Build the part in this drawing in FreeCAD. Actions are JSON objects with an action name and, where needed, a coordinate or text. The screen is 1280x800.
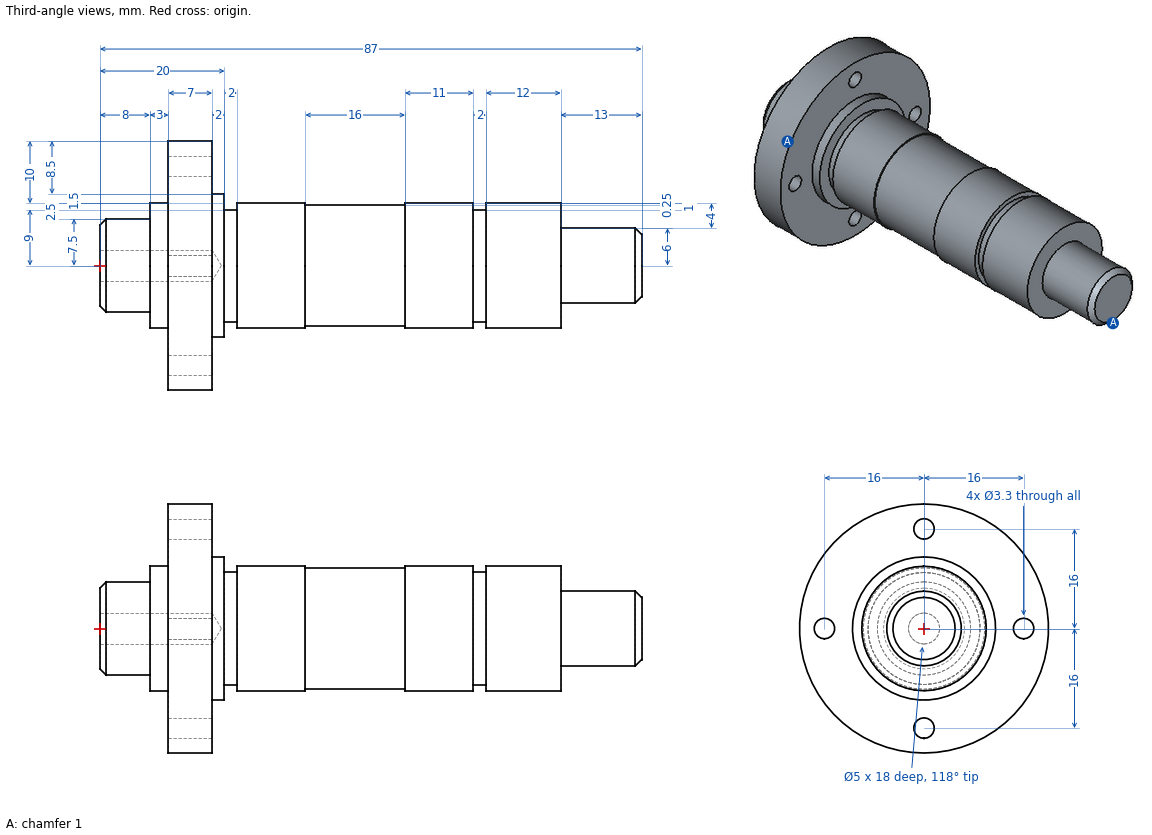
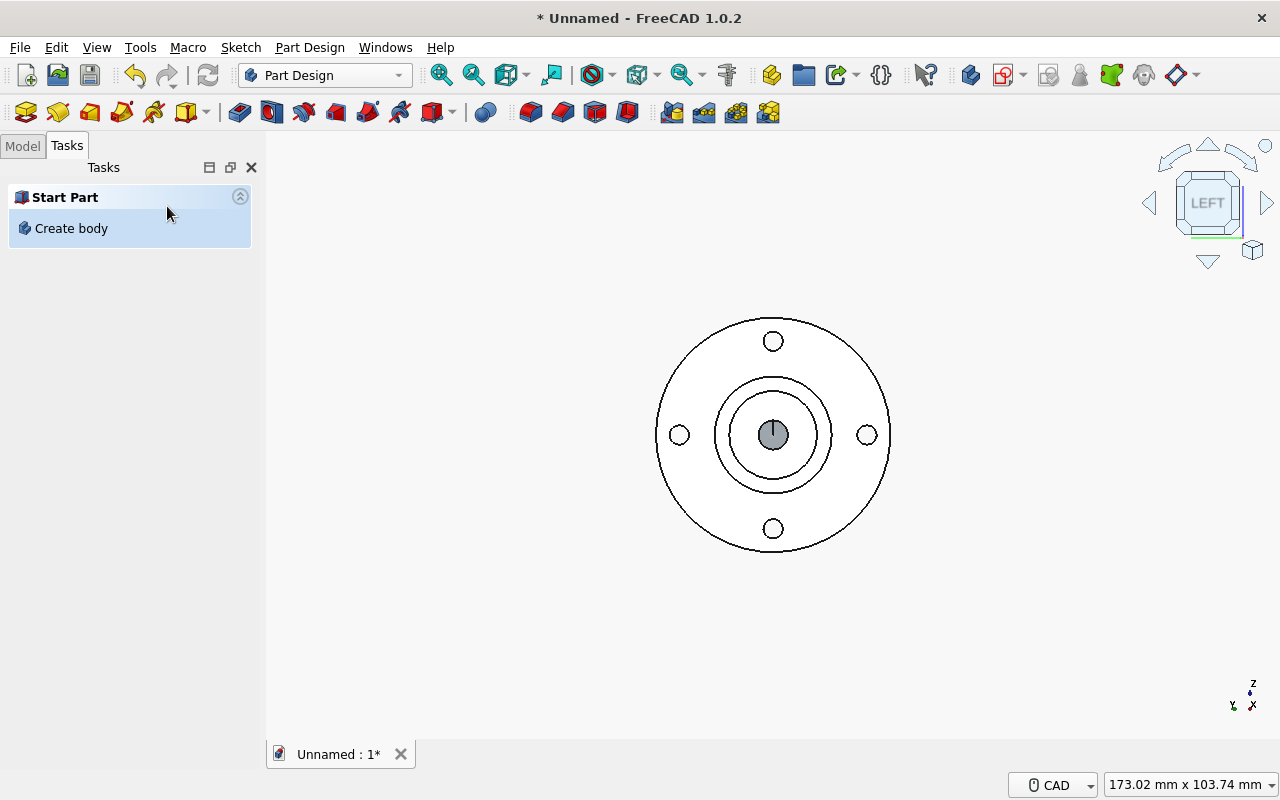
{"action": "left_click", "coordinate": [442, 76]}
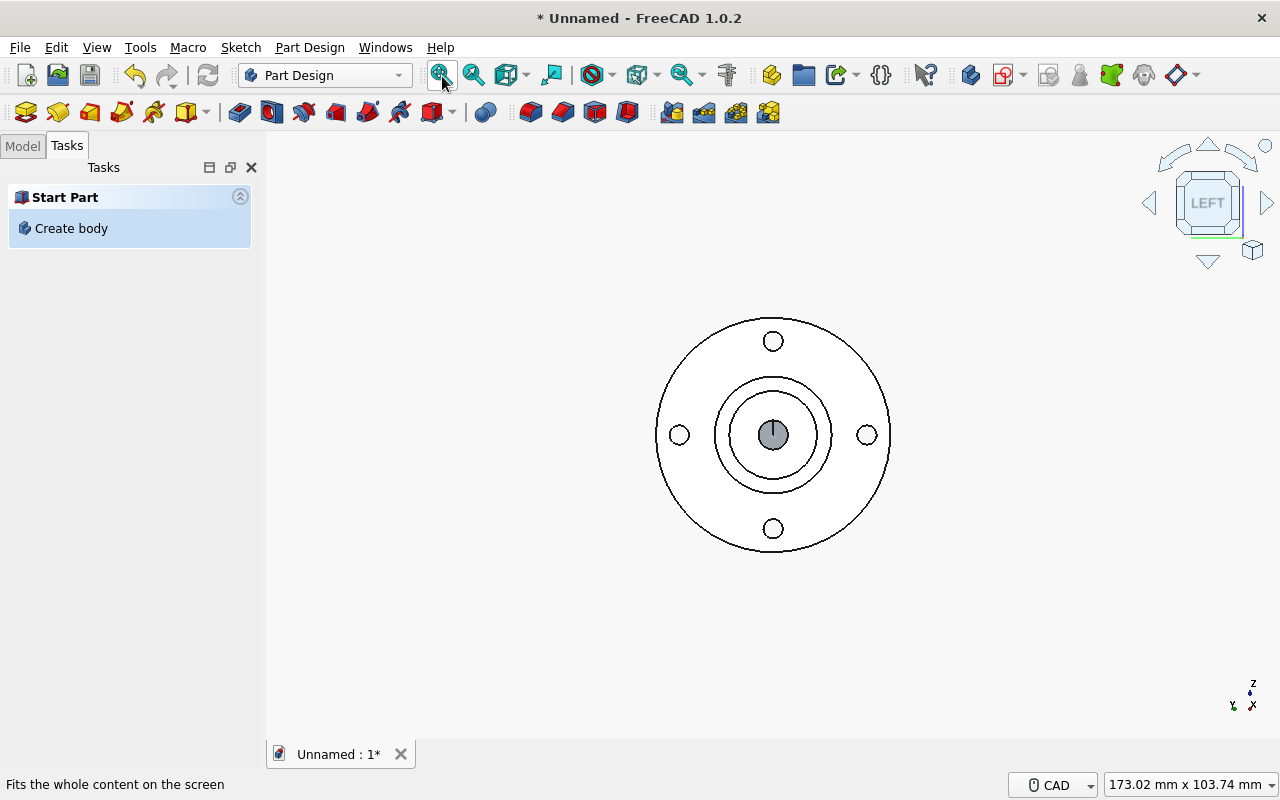
{"action": "left_click", "coordinate": [1004, 76]}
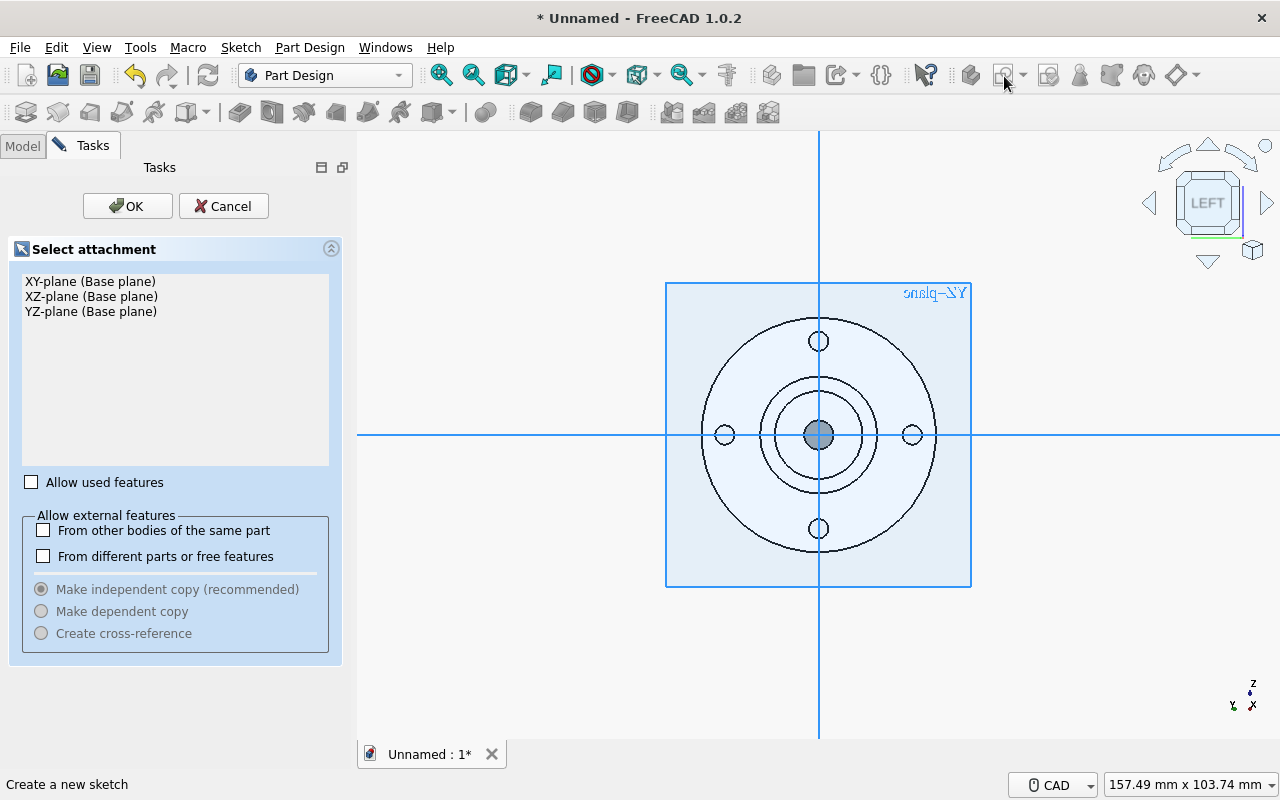
{"action": "left_click", "coordinate": [82, 282]}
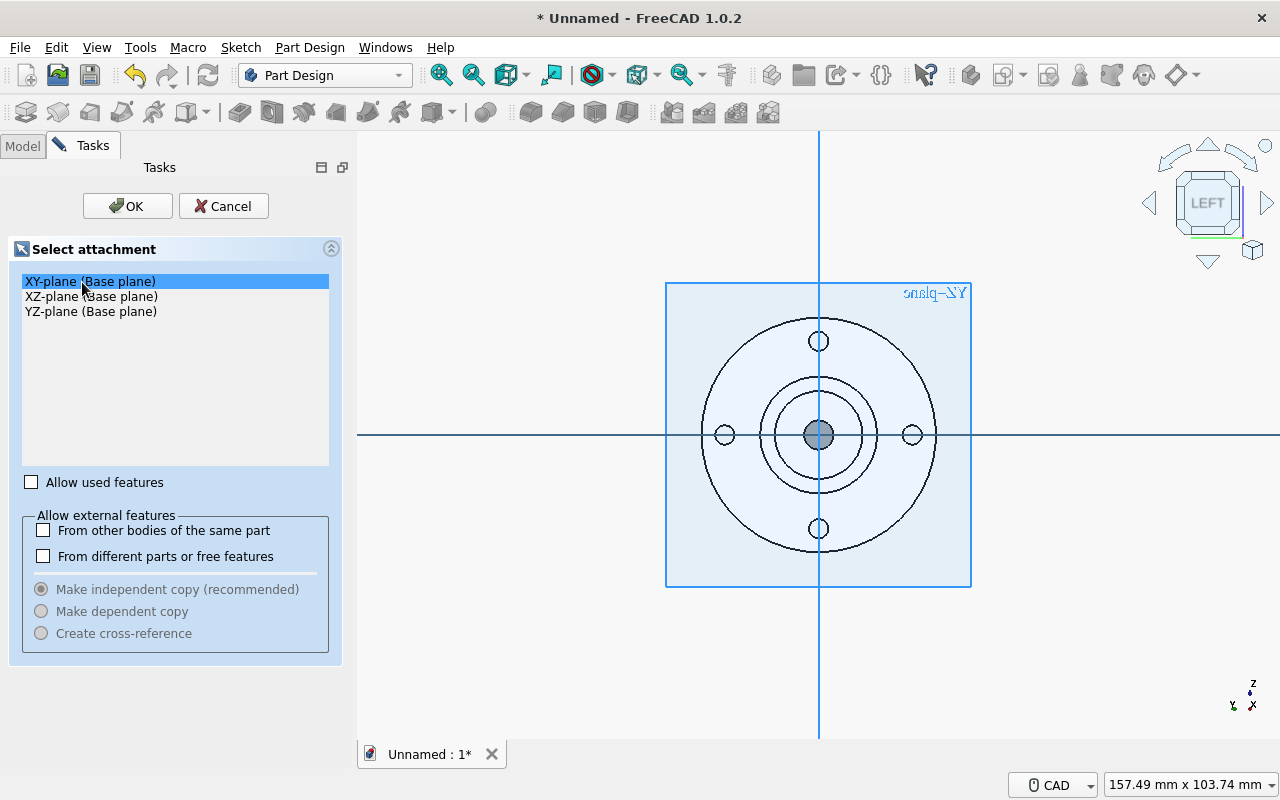
{"action": "left_click", "coordinate": [128, 206]}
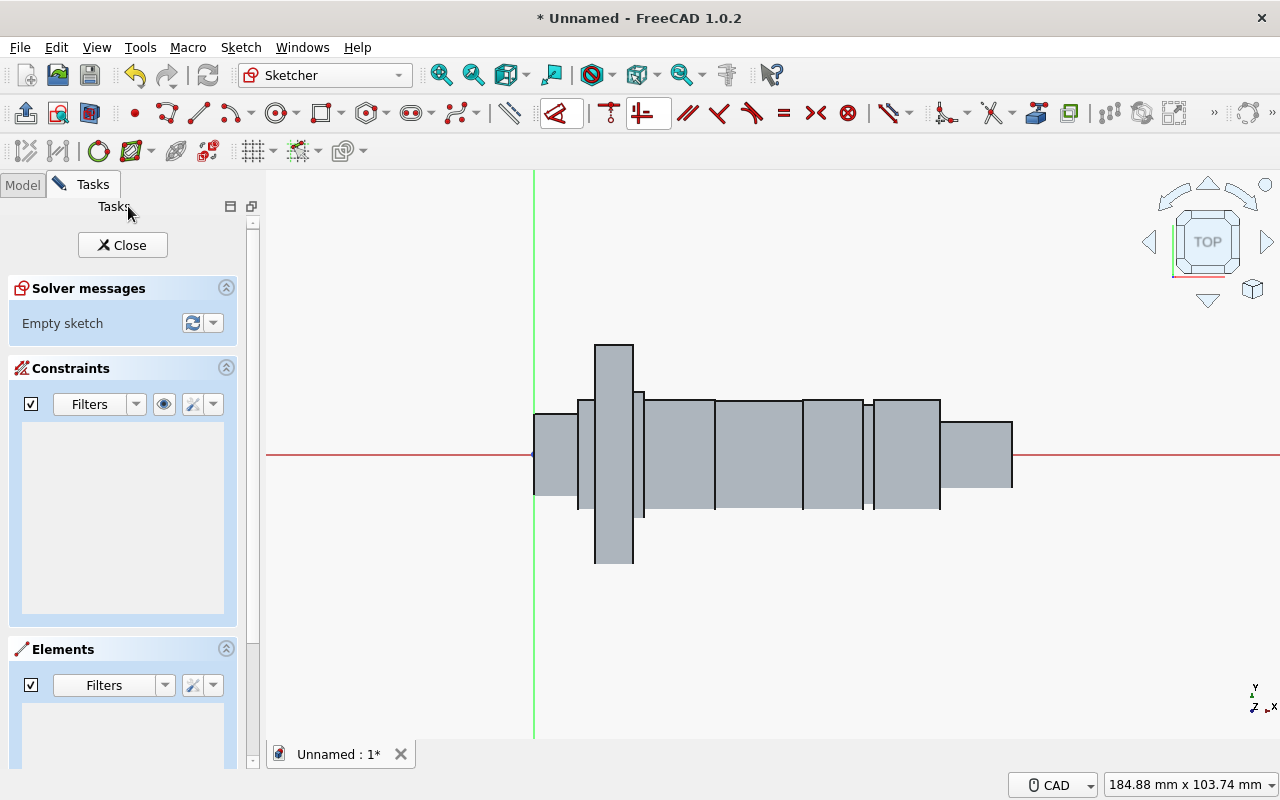
{"action": "left_click", "coordinate": [90, 114]}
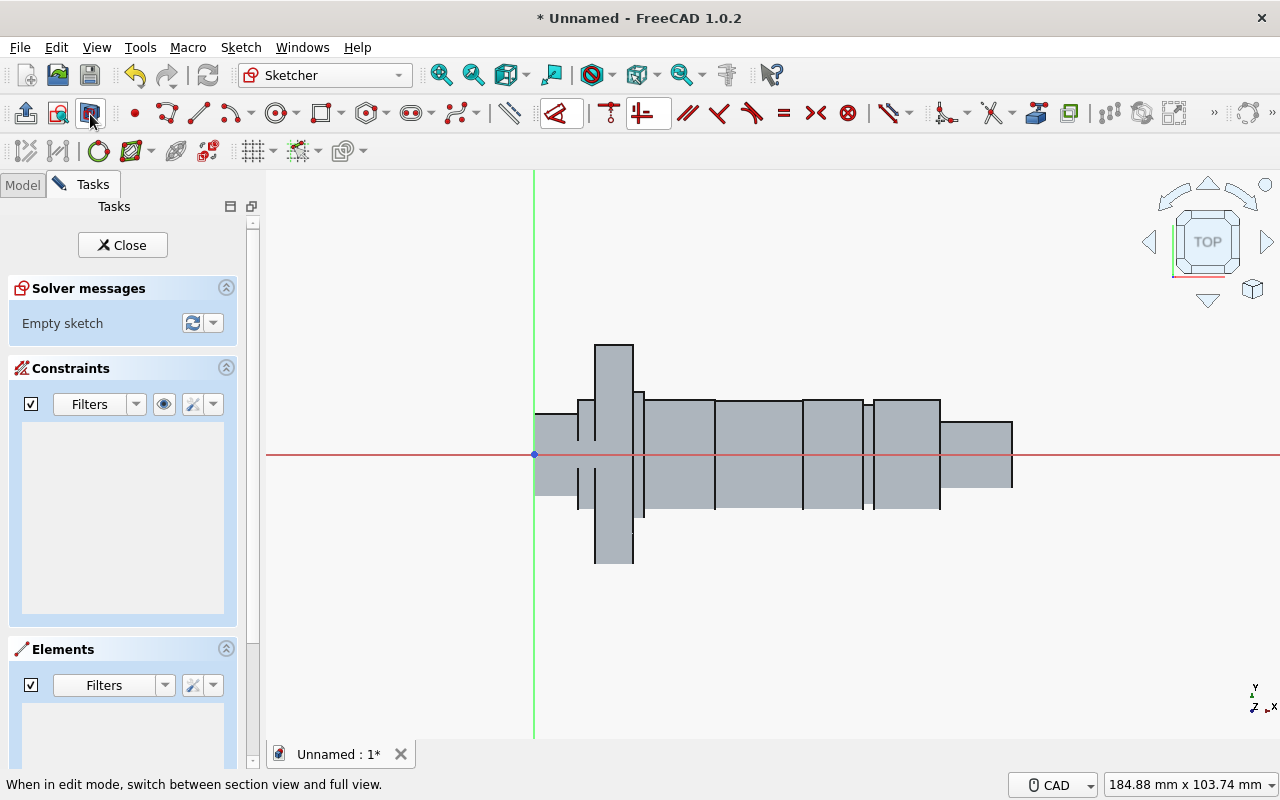
{"action": "scroll", "coordinate": [647, 400], "scroll_direction": "up", "scroll_amount": 15}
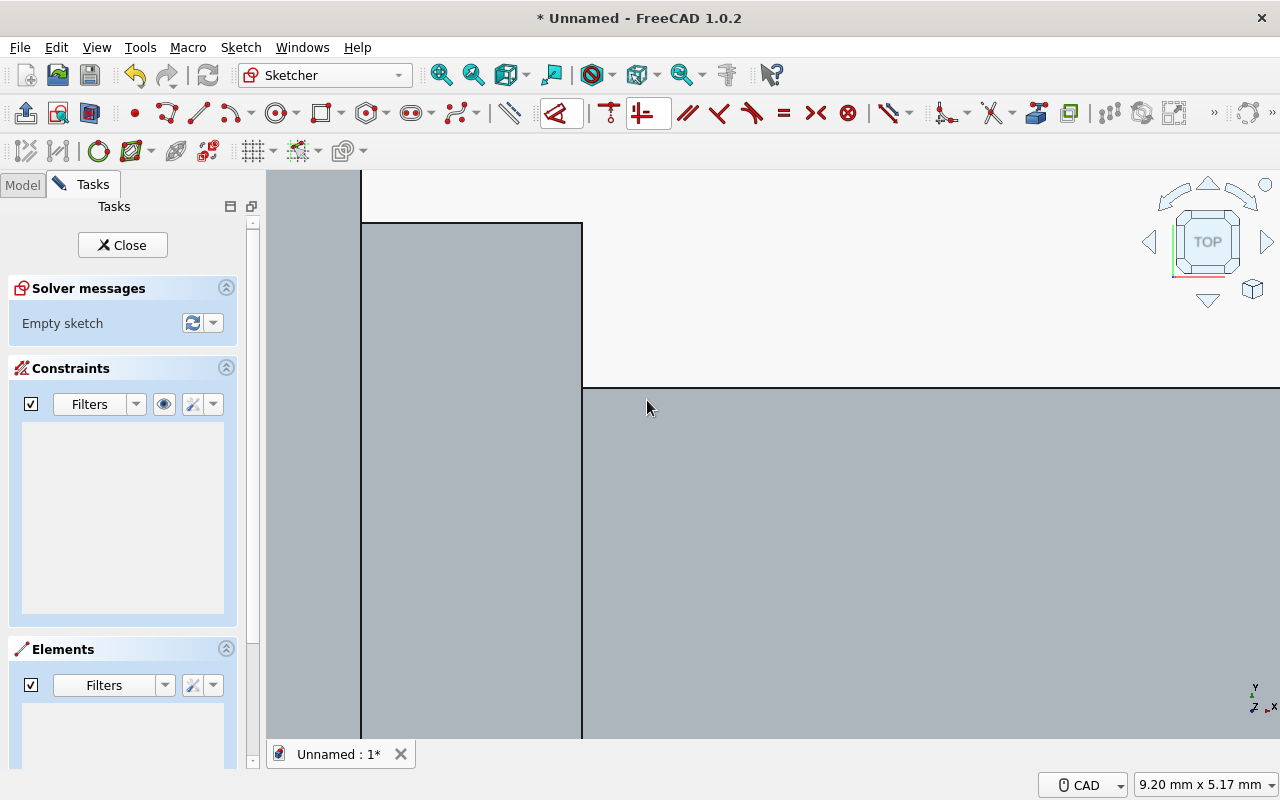
{"action": "scroll", "coordinate": [685, 437], "scroll_direction": "up", "scroll_amount": 5}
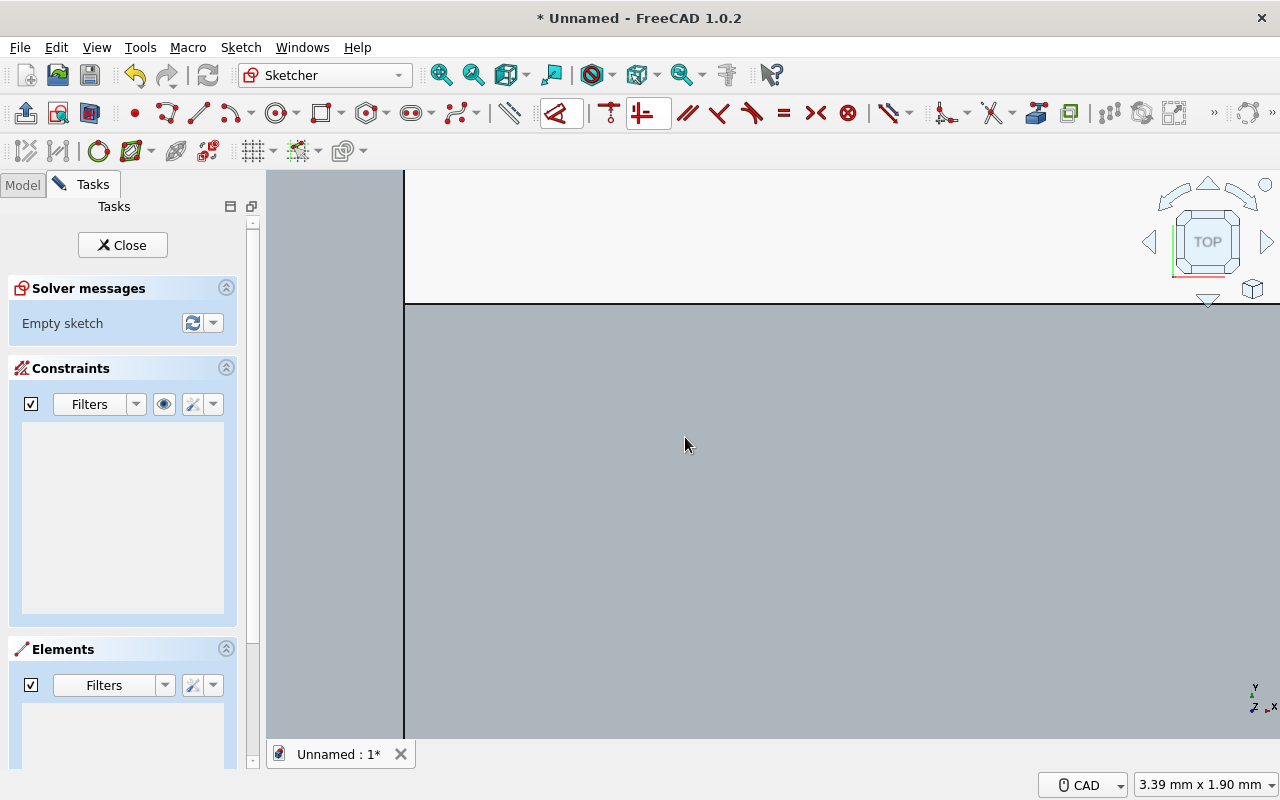
{"action": "left_click", "coordinate": [322, 114]}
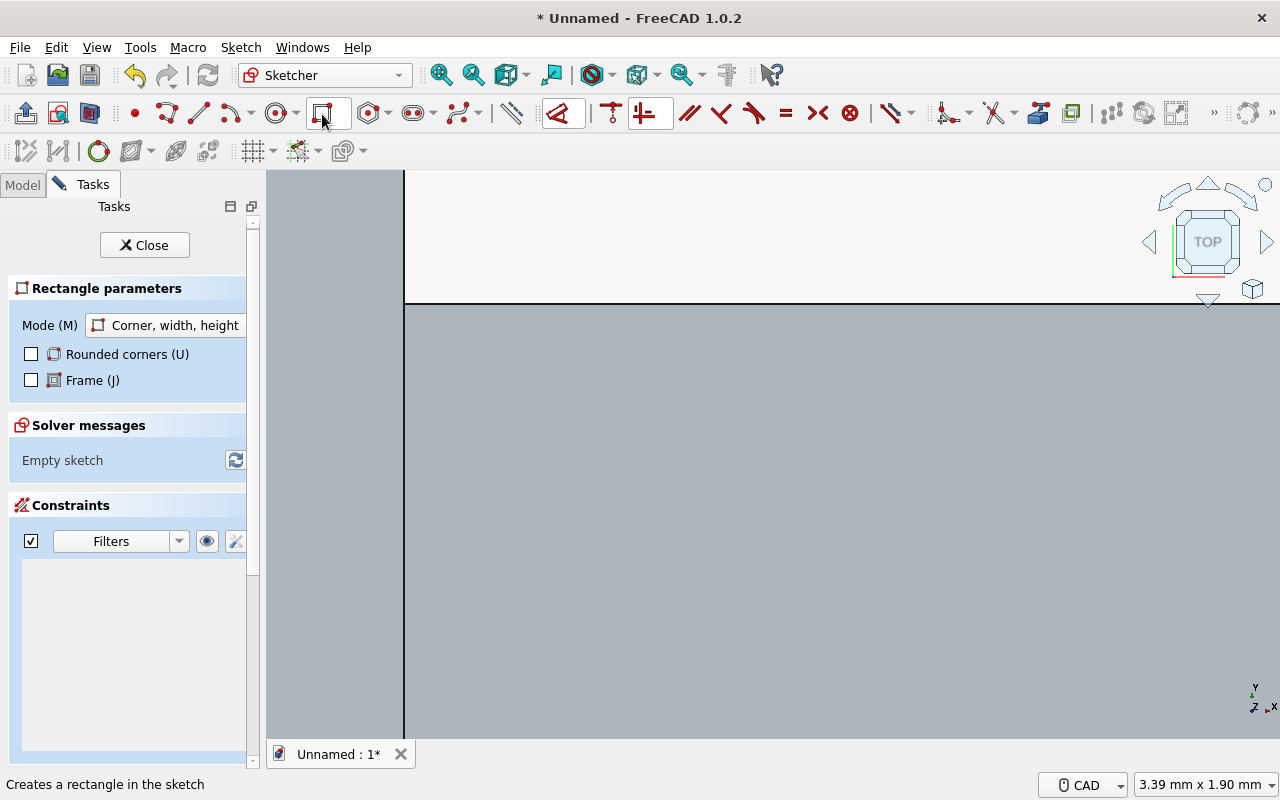
{"action": "left_click", "coordinate": [404, 304]}
{"action": "mouse_move", "coordinate": [1003, 603]}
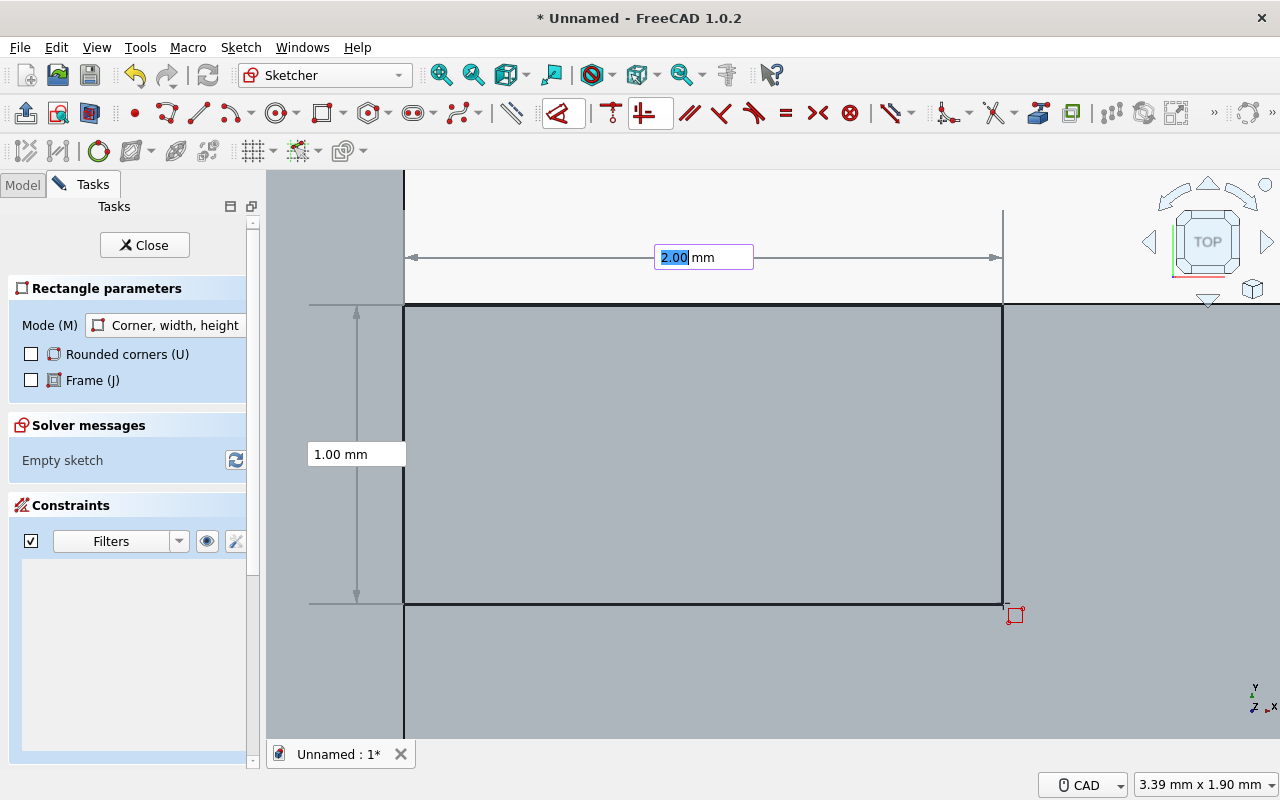
{"action": "type", "text": "2"}
{"action": "key", "text": "Tab"}
{"action": "type", "text": "1"}
{"action": "key", "text": "Return"}
{"action": "key", "text": "Escape"}